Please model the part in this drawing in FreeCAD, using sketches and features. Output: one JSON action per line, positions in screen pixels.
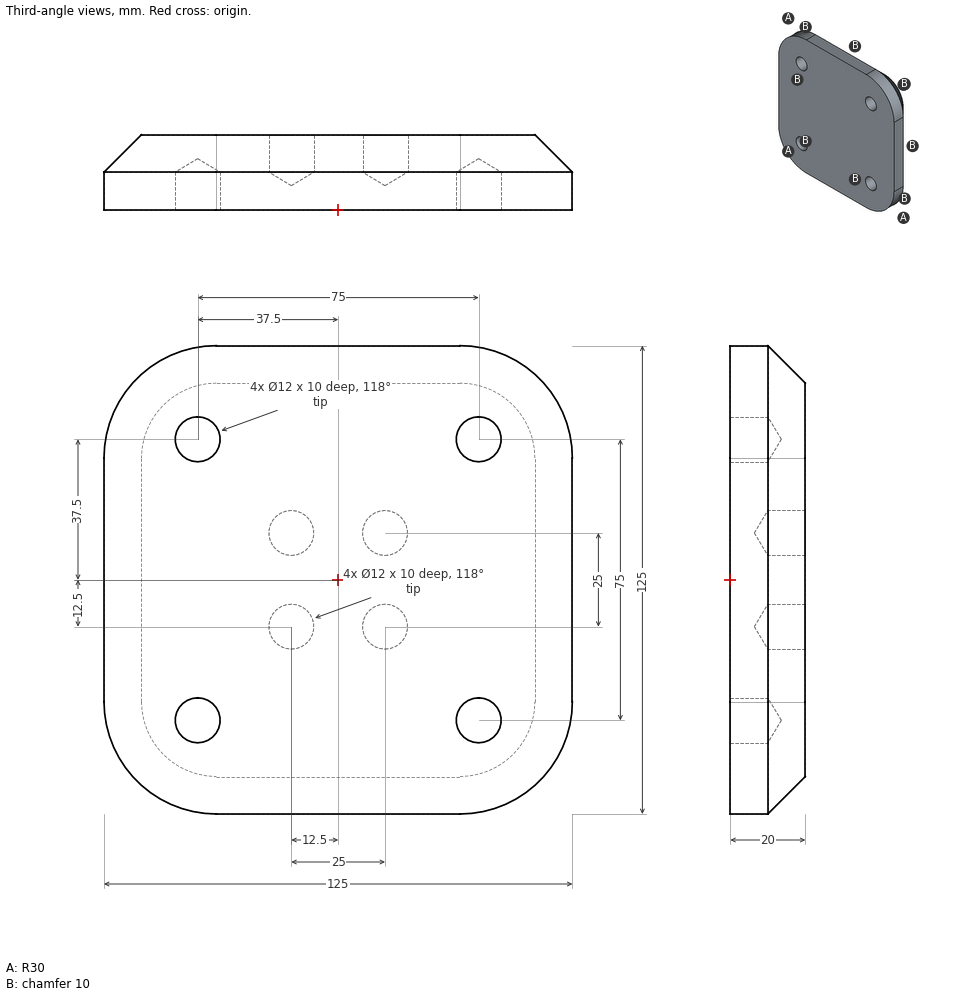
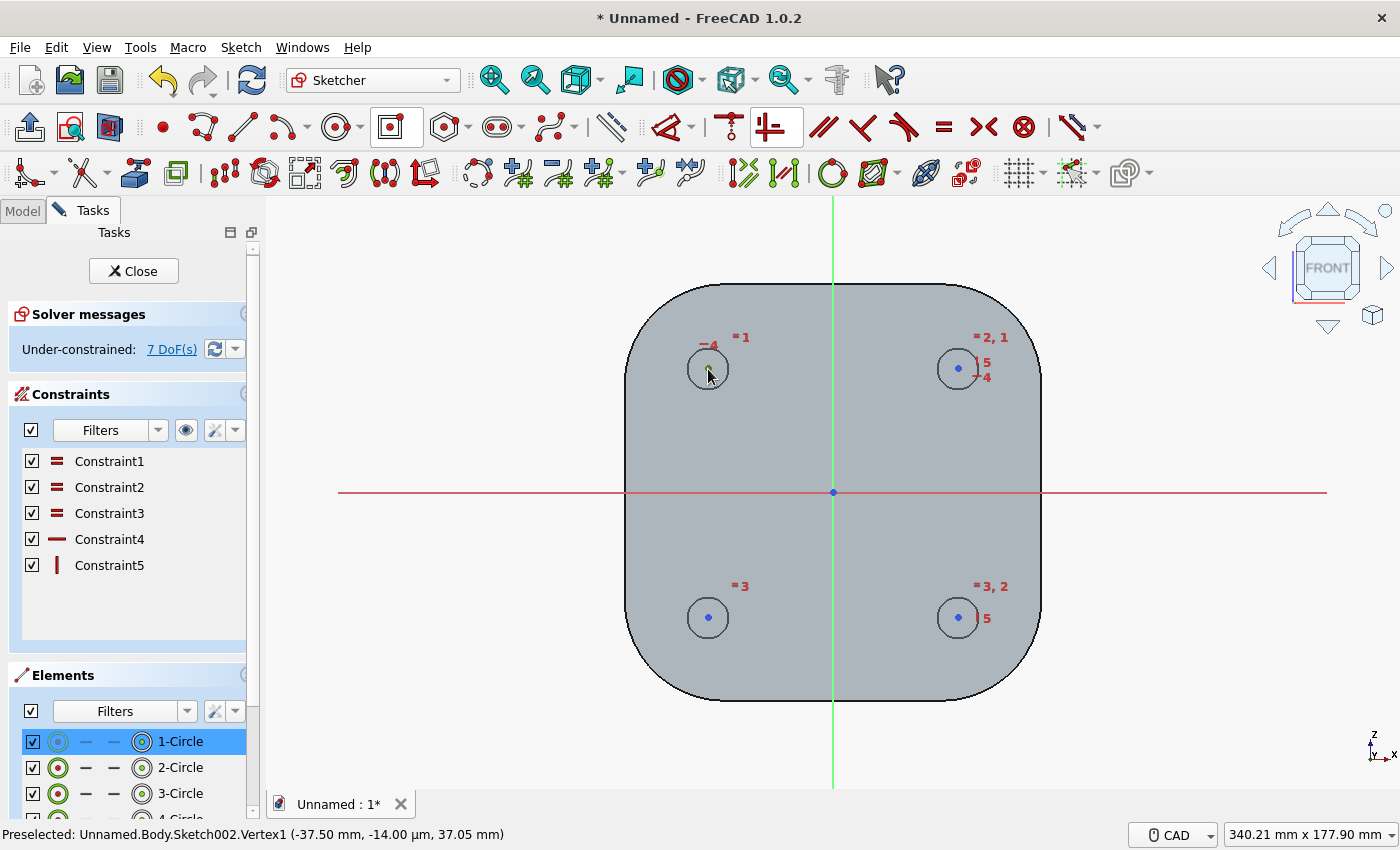
{"action": "left_click", "coordinate": [708, 618]}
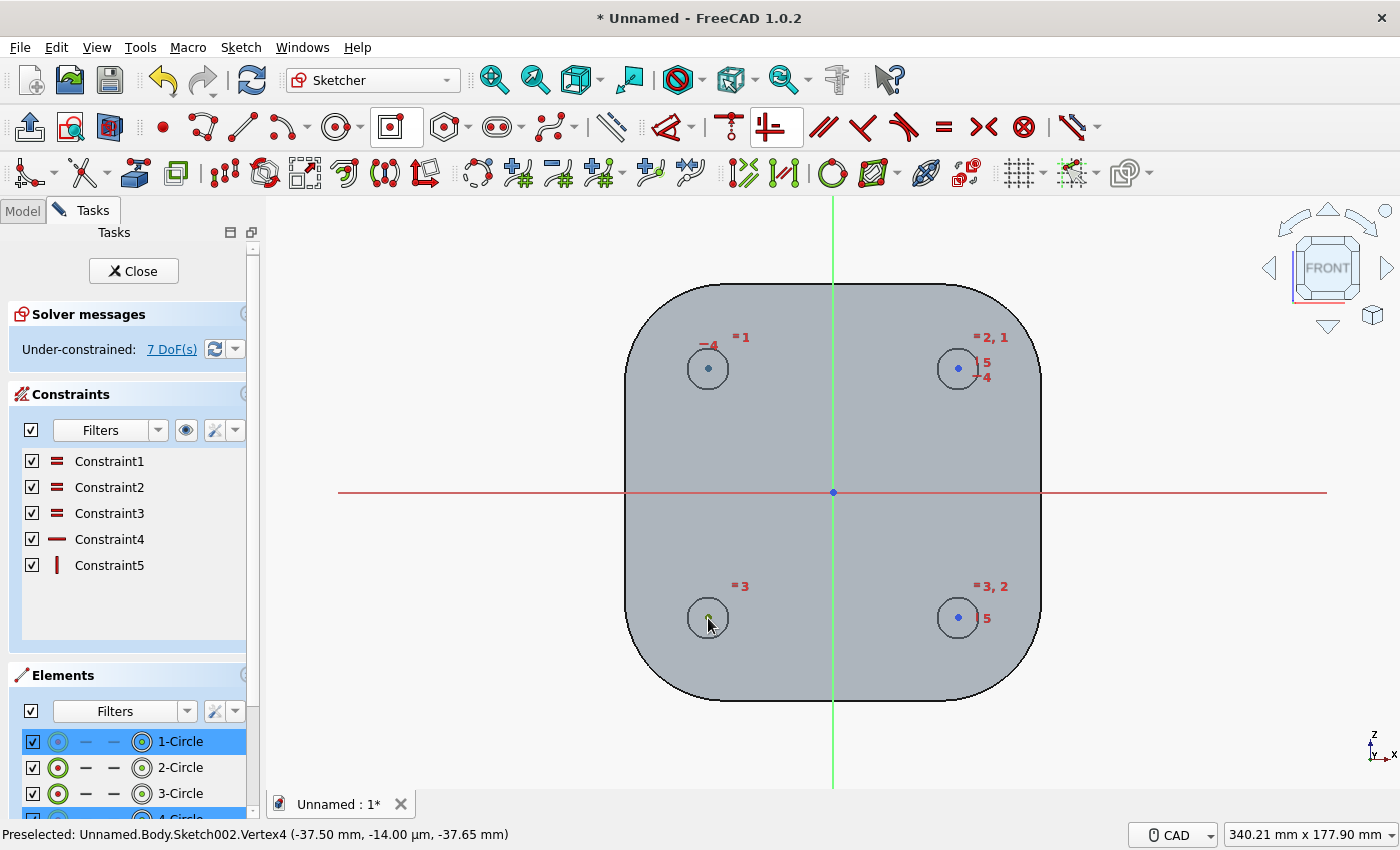
{"action": "key", "text": "v"}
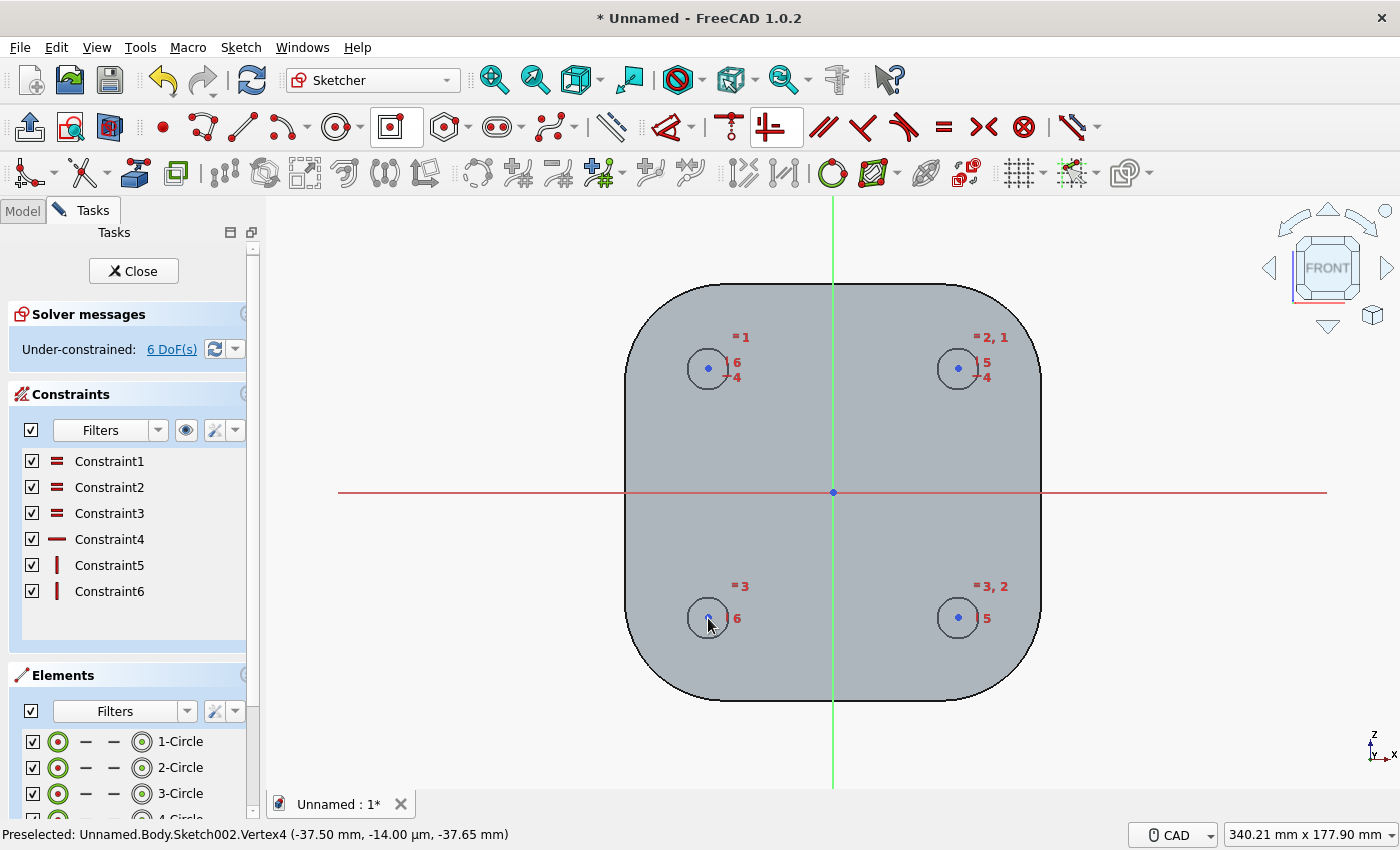
{"action": "left_click", "coordinate": [958, 618]}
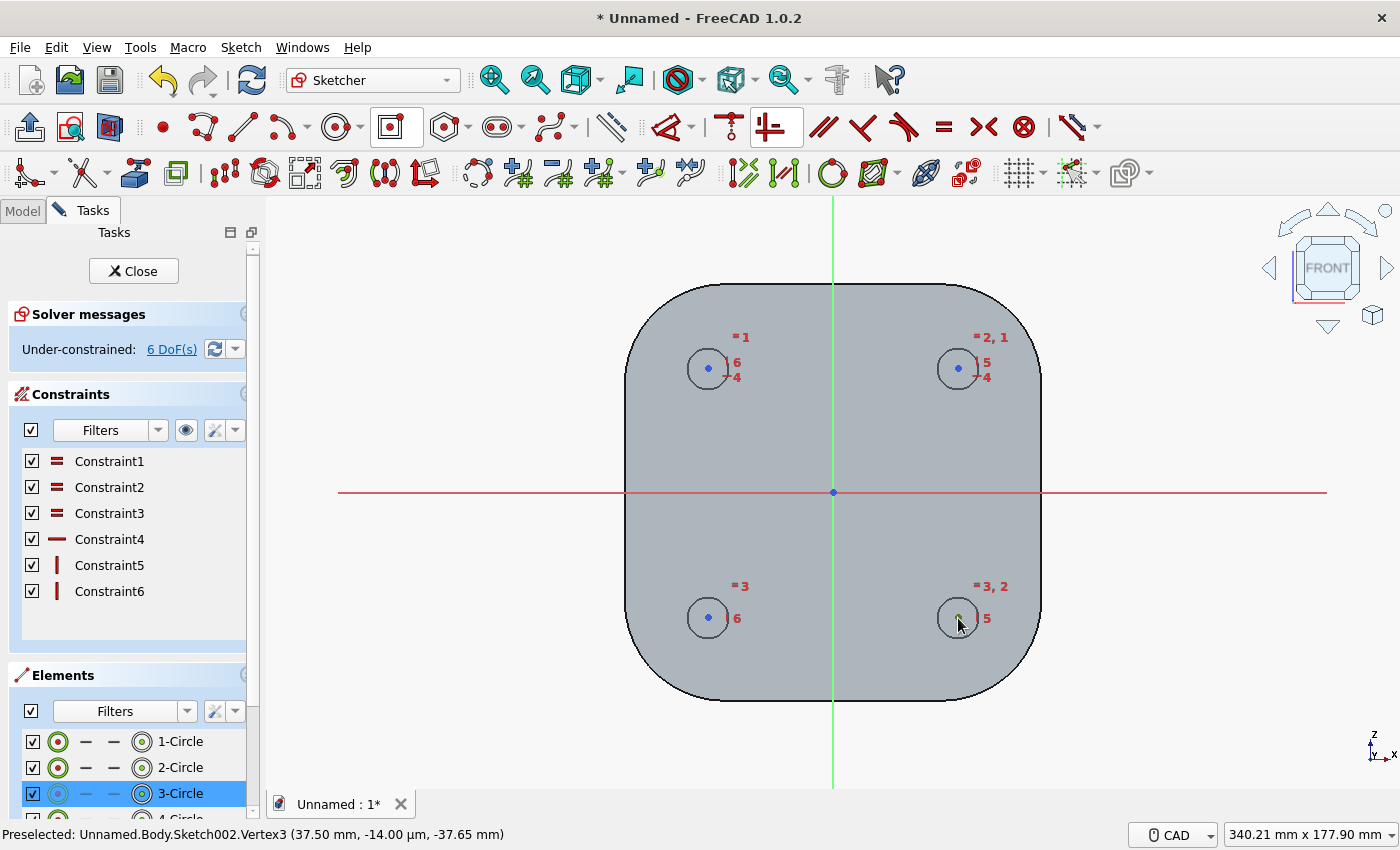
{"action": "left_click", "coordinate": [708, 618]}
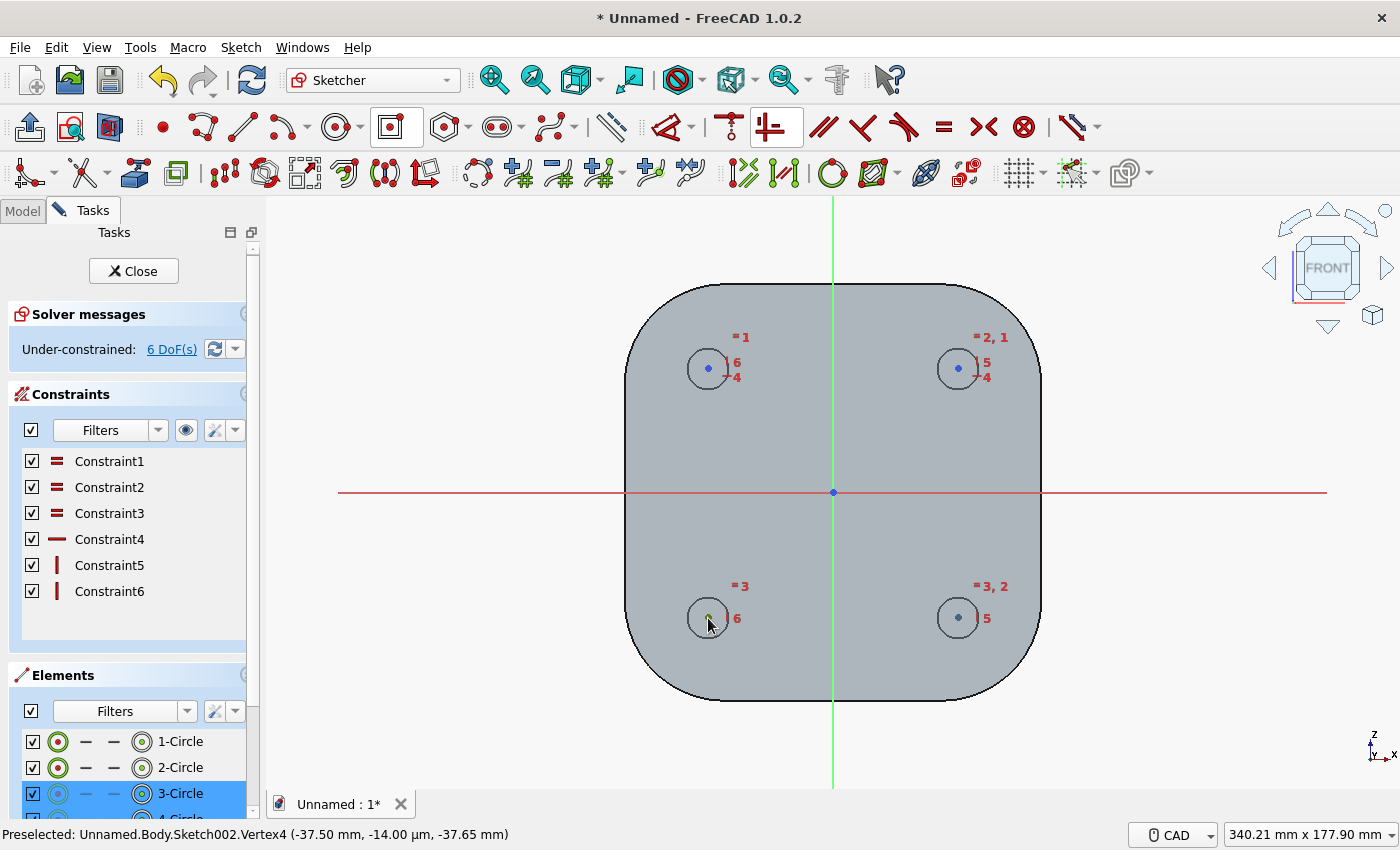
{"action": "key", "text": "h"}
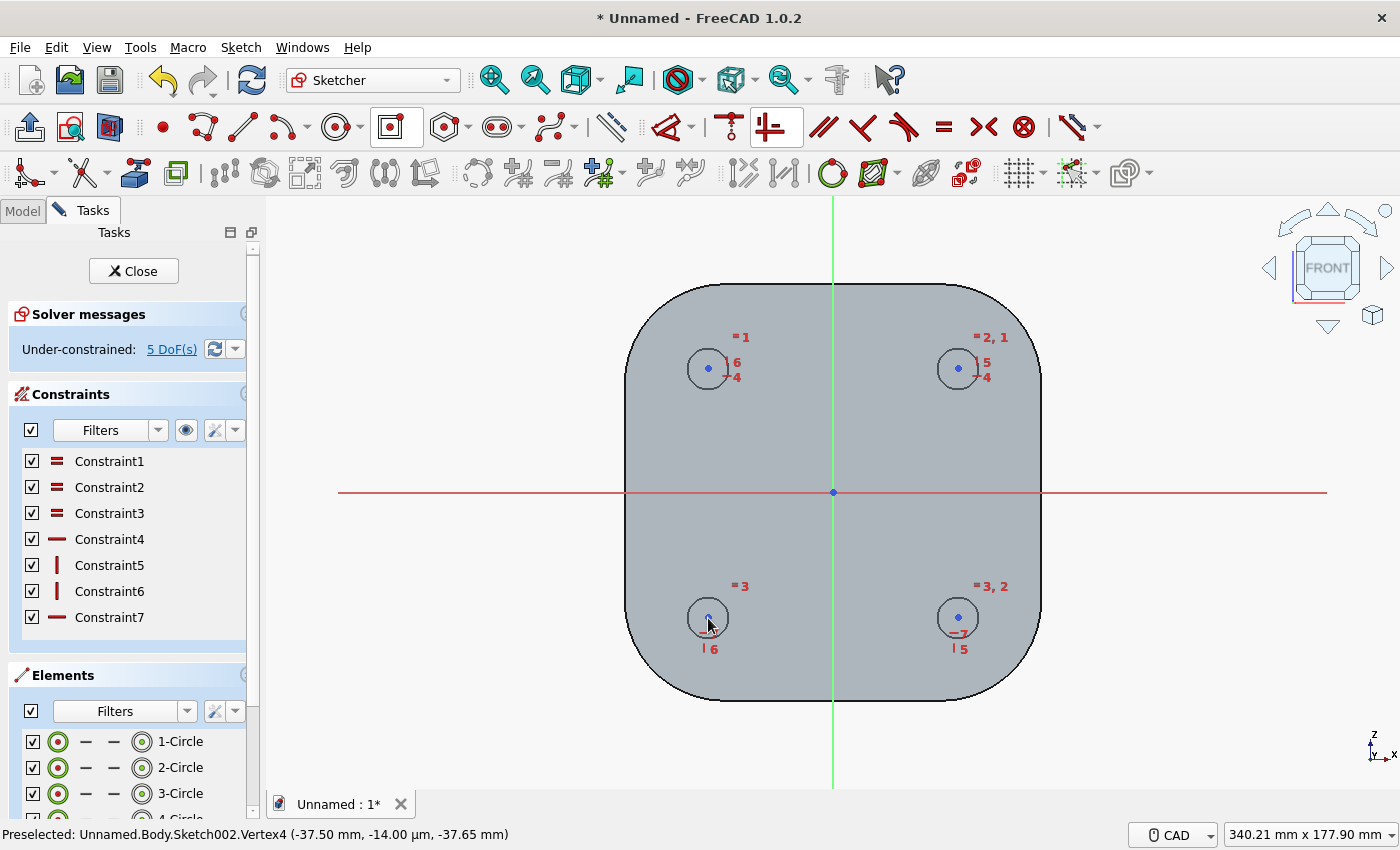
{"action": "key", "text": "d"}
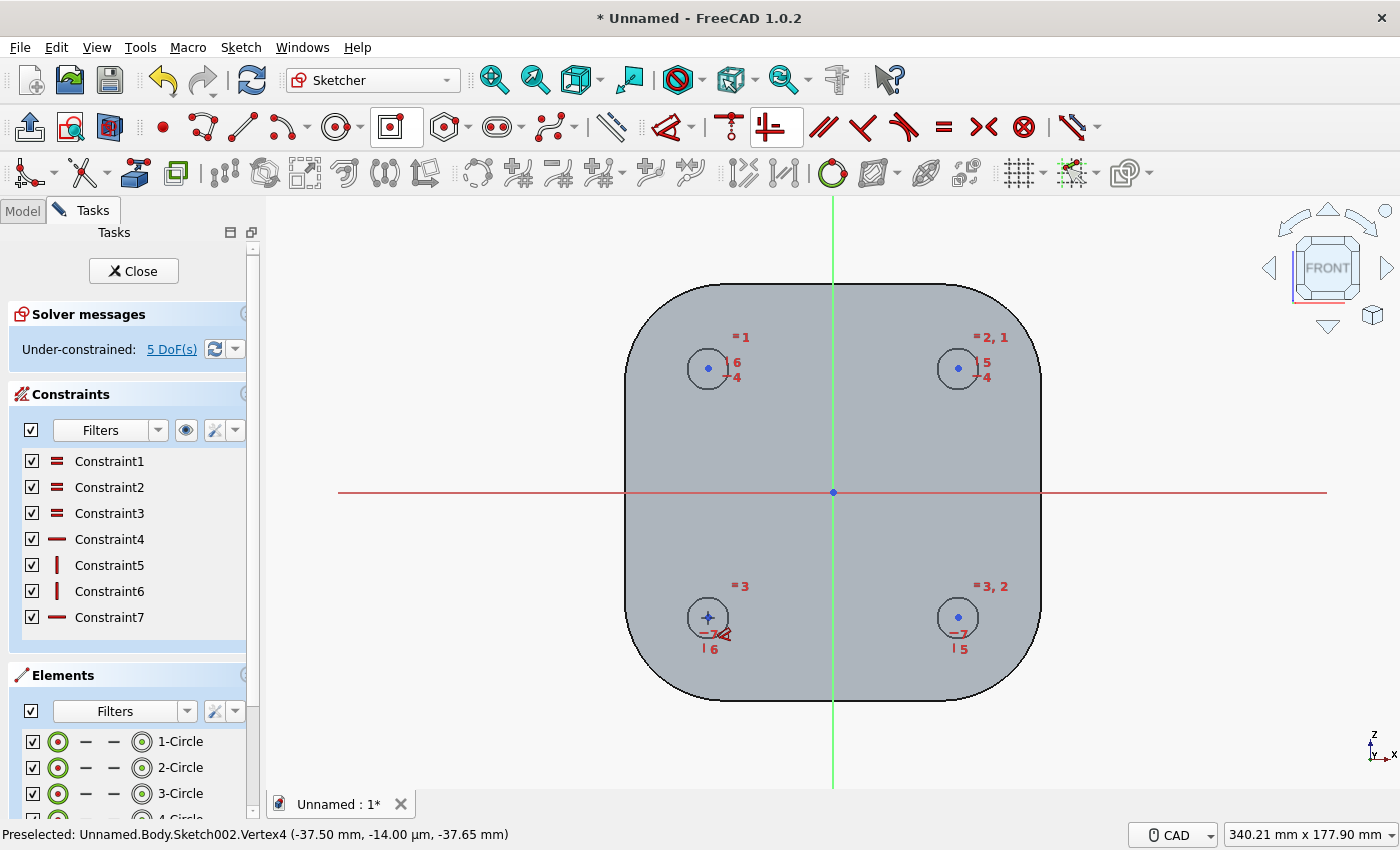
{"action": "left_click", "coordinate": [722, 354]}
{"action": "left_click", "coordinate": [744, 331]}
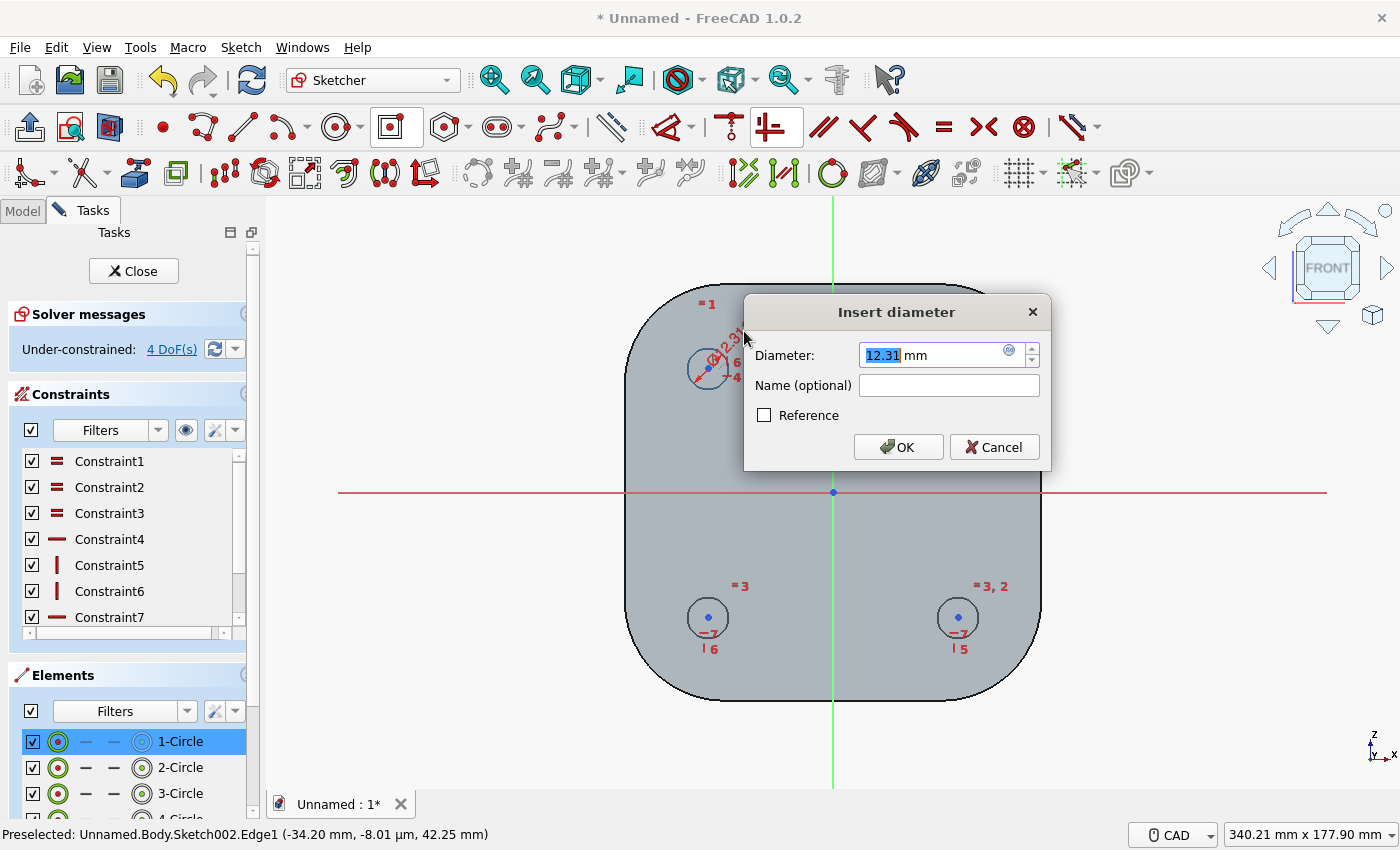
{"action": "type", "text": "12"}
{"action": "key", "text": "Return"}